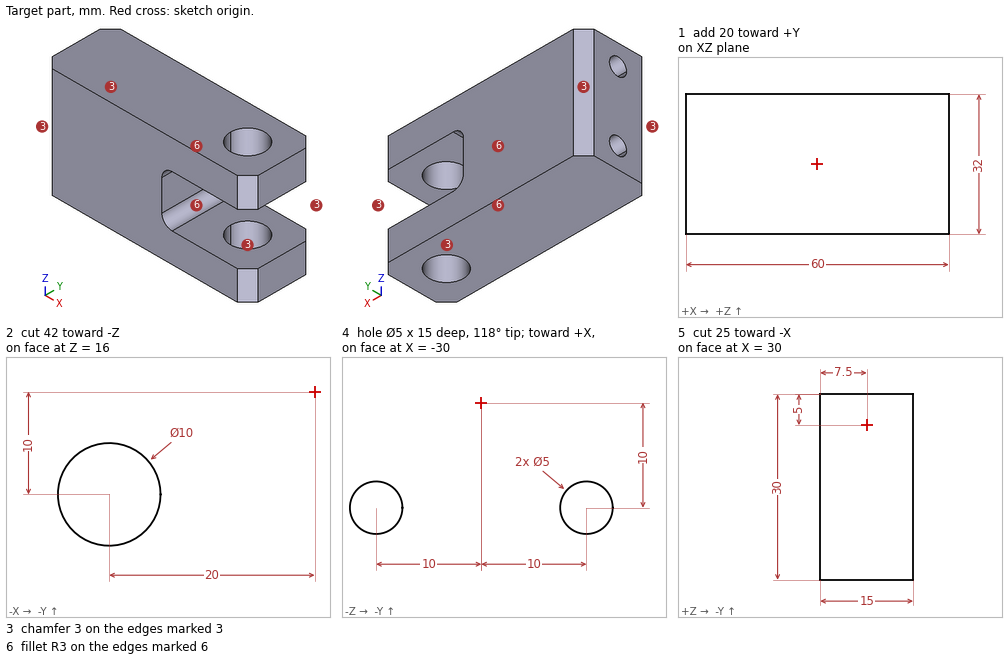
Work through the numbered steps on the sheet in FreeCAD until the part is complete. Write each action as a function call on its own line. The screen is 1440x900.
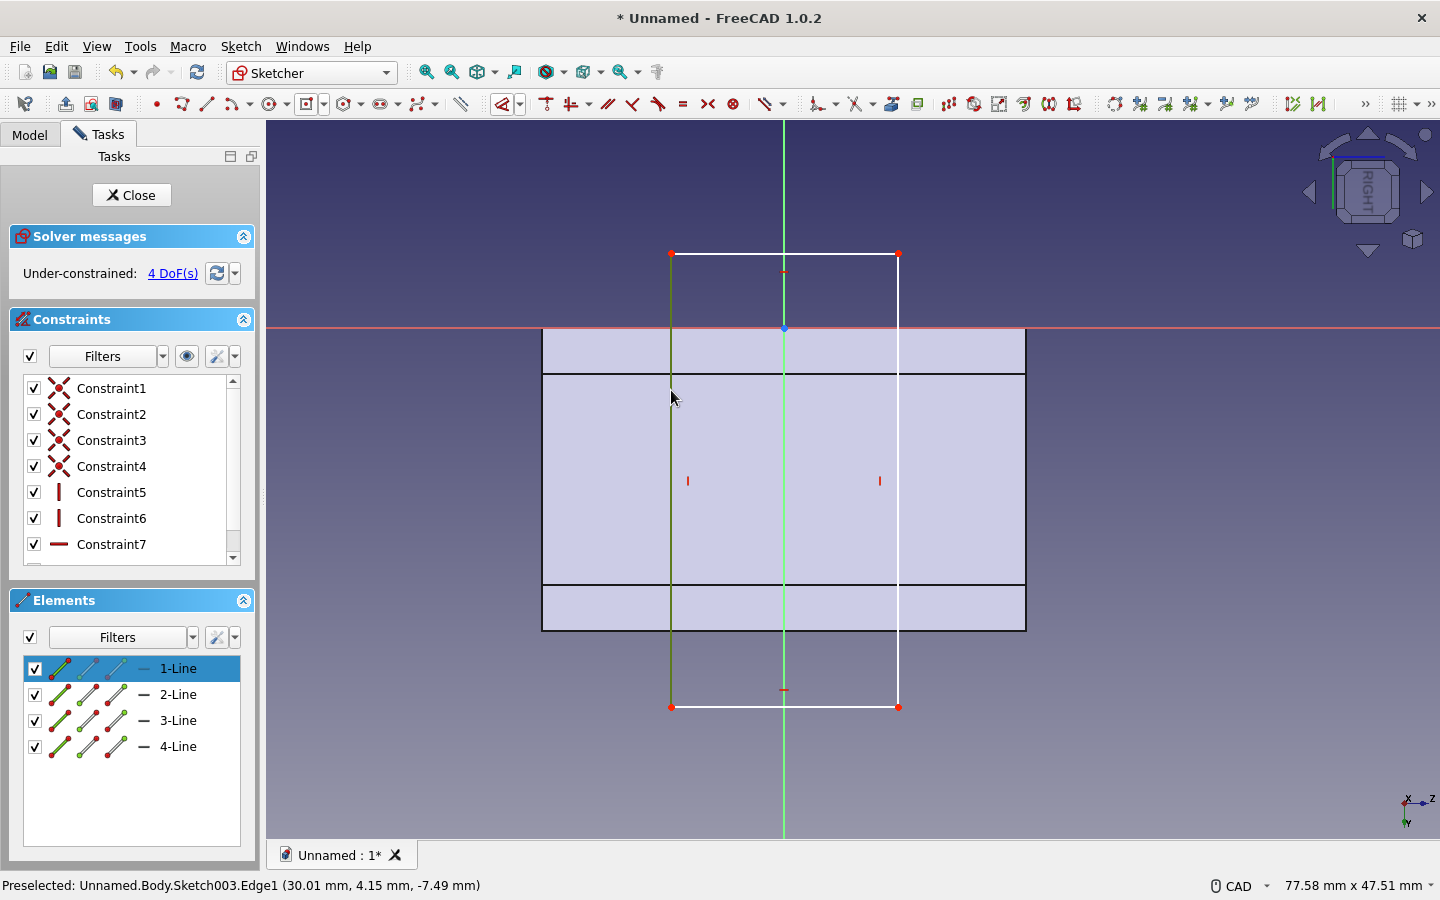
key(i)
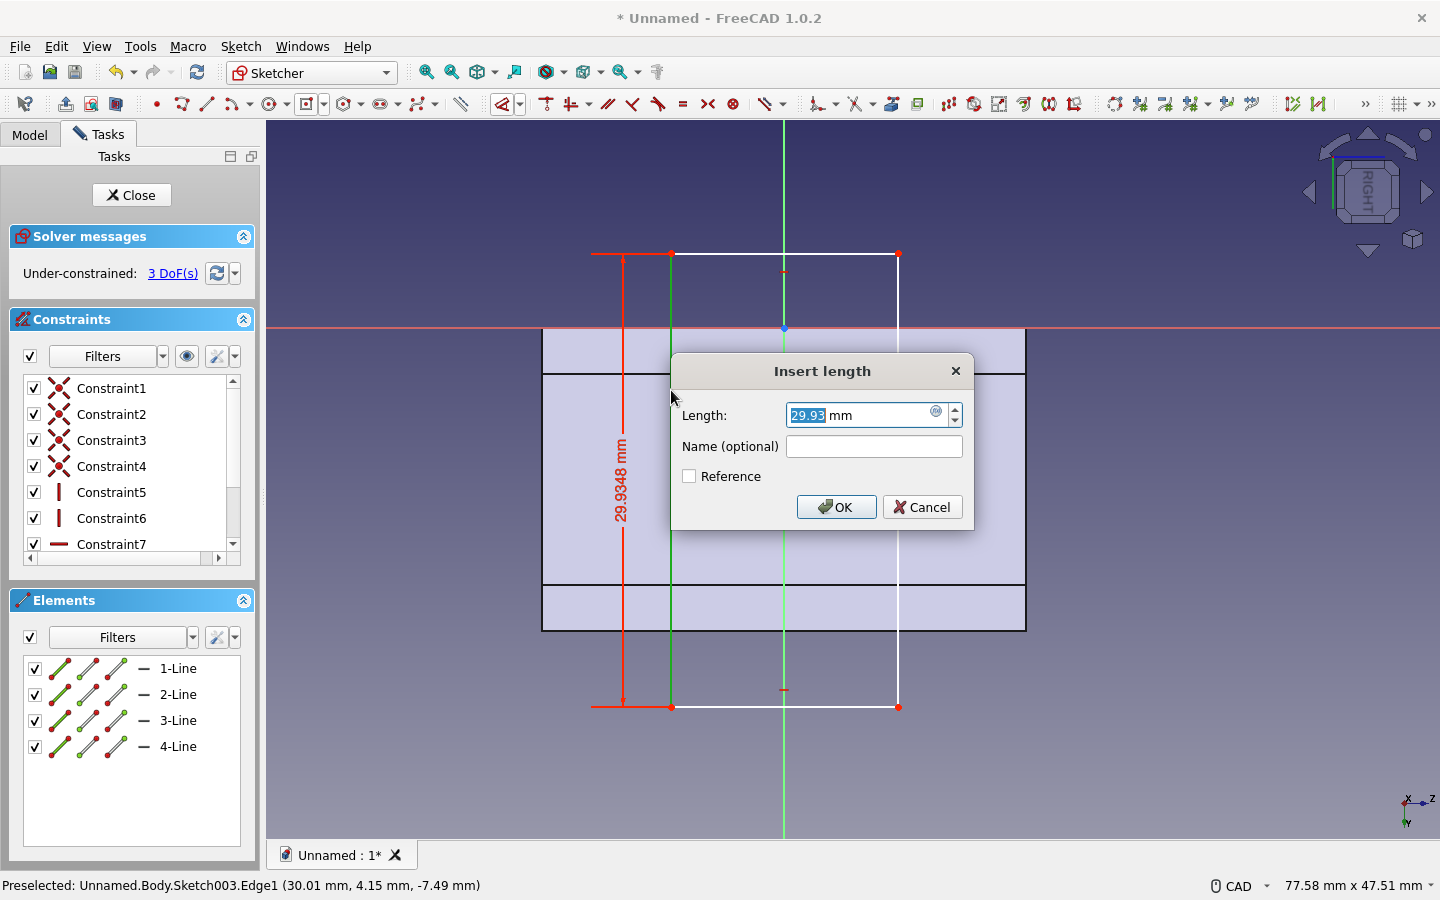
text(30)
key(Return)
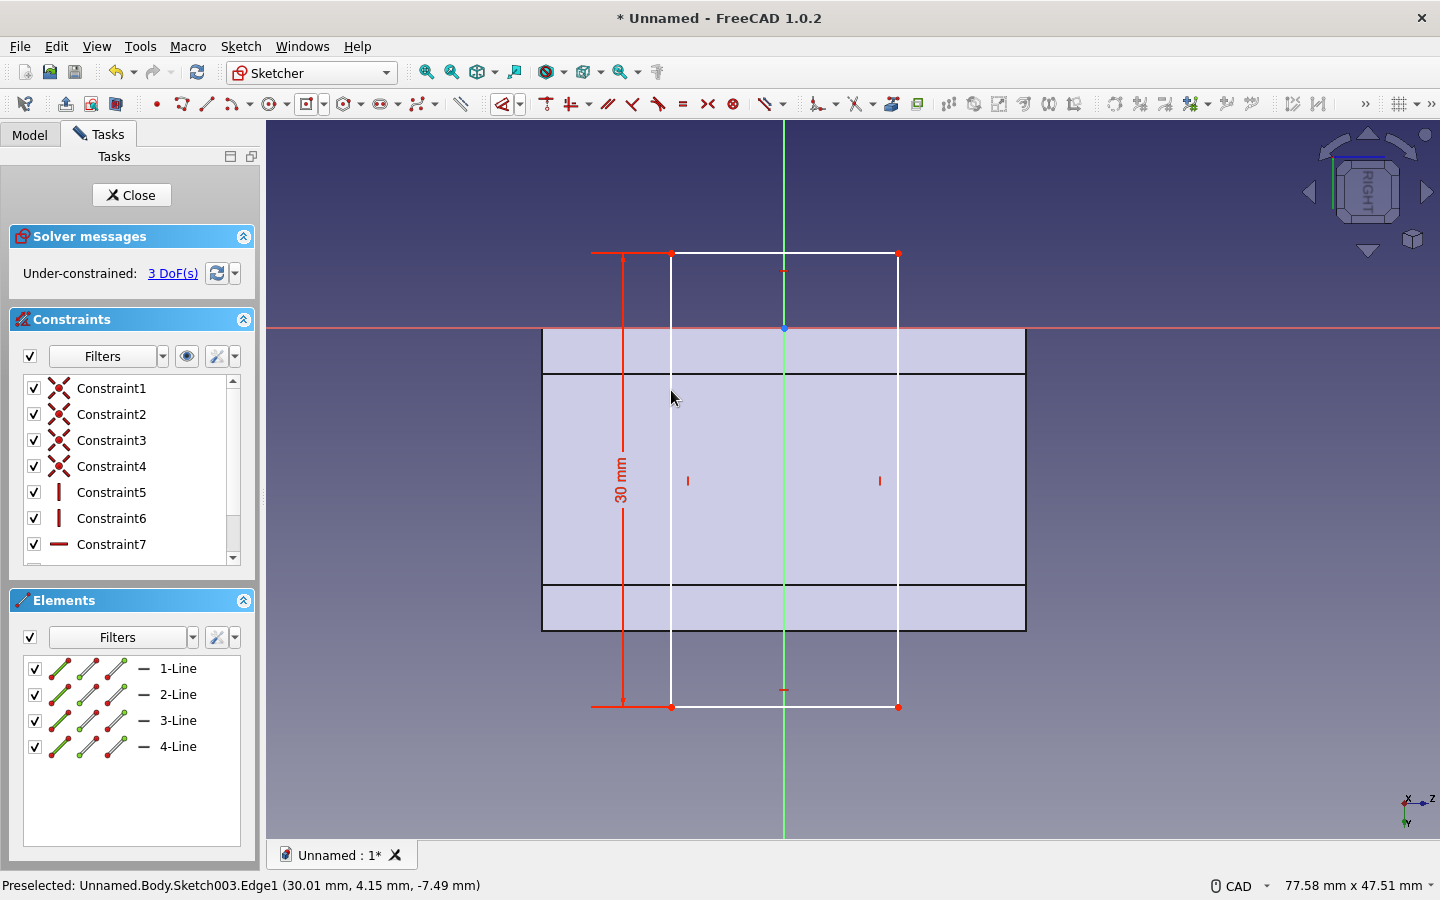
click(739, 707)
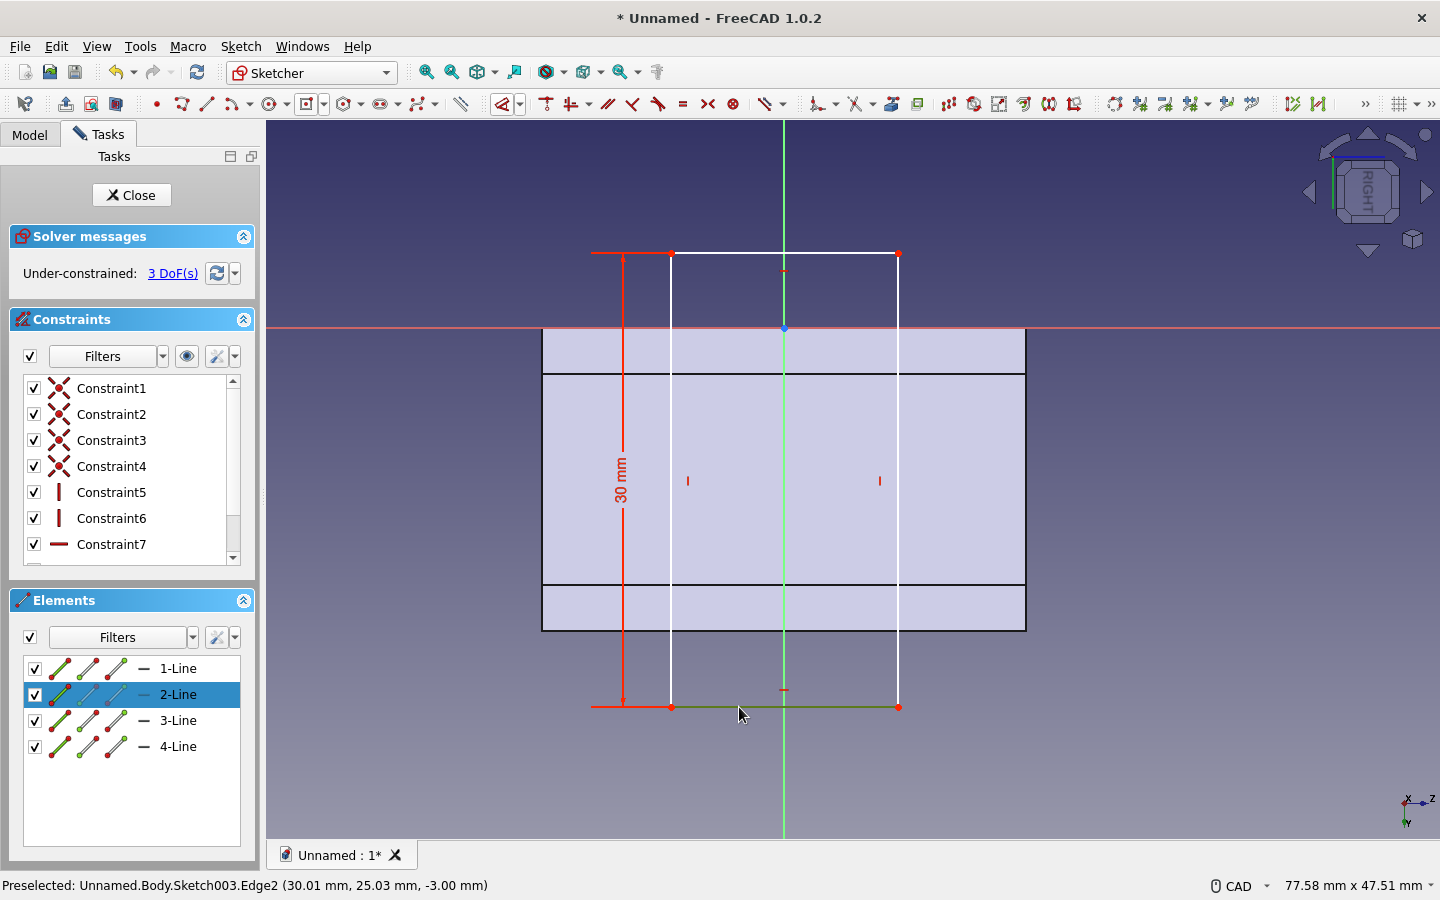
click(520, 104)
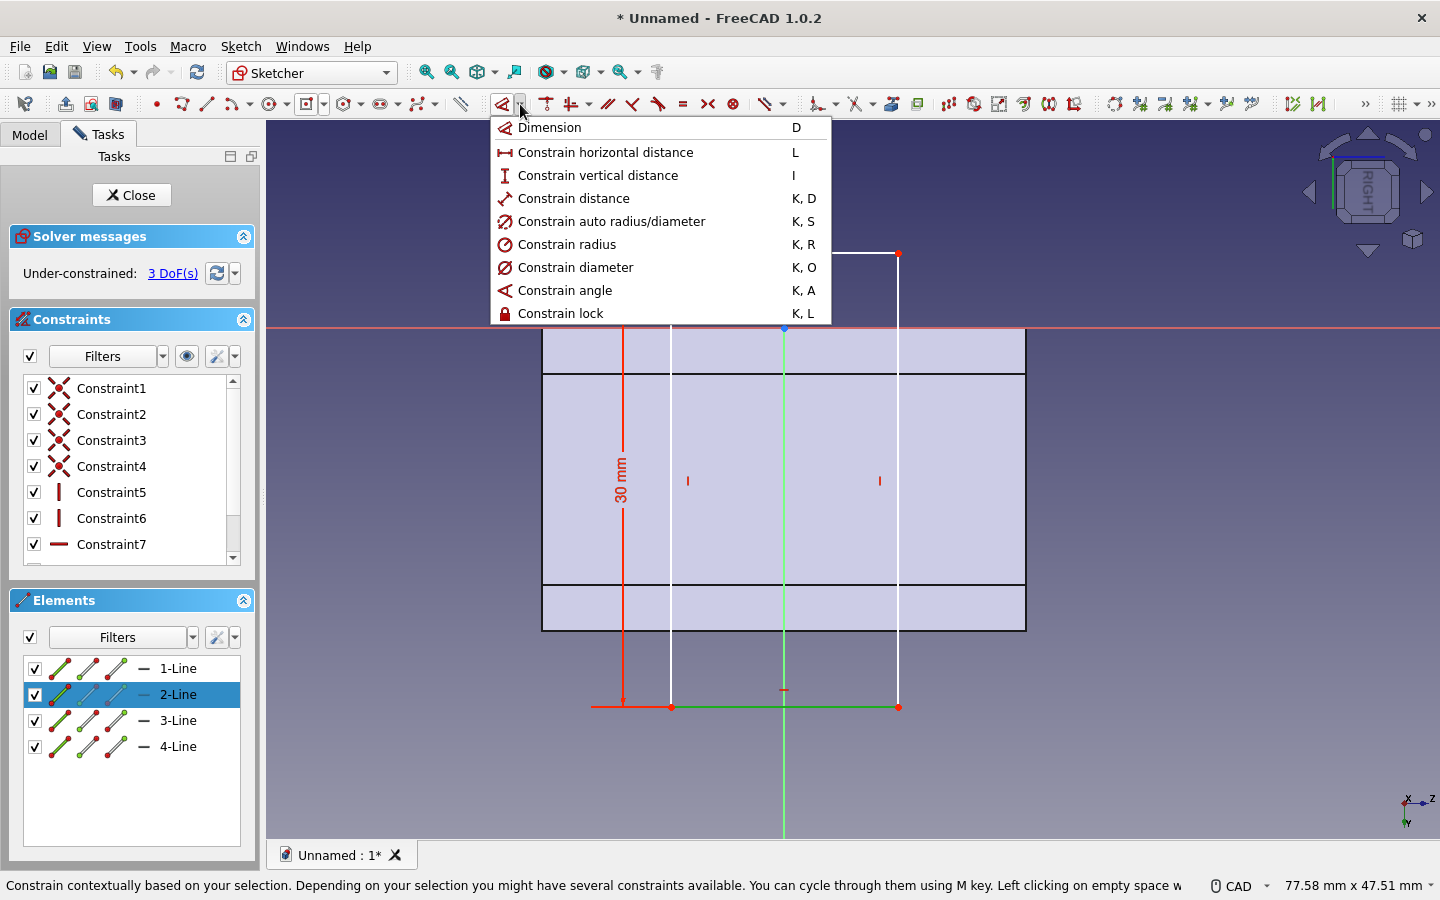
click(661, 152)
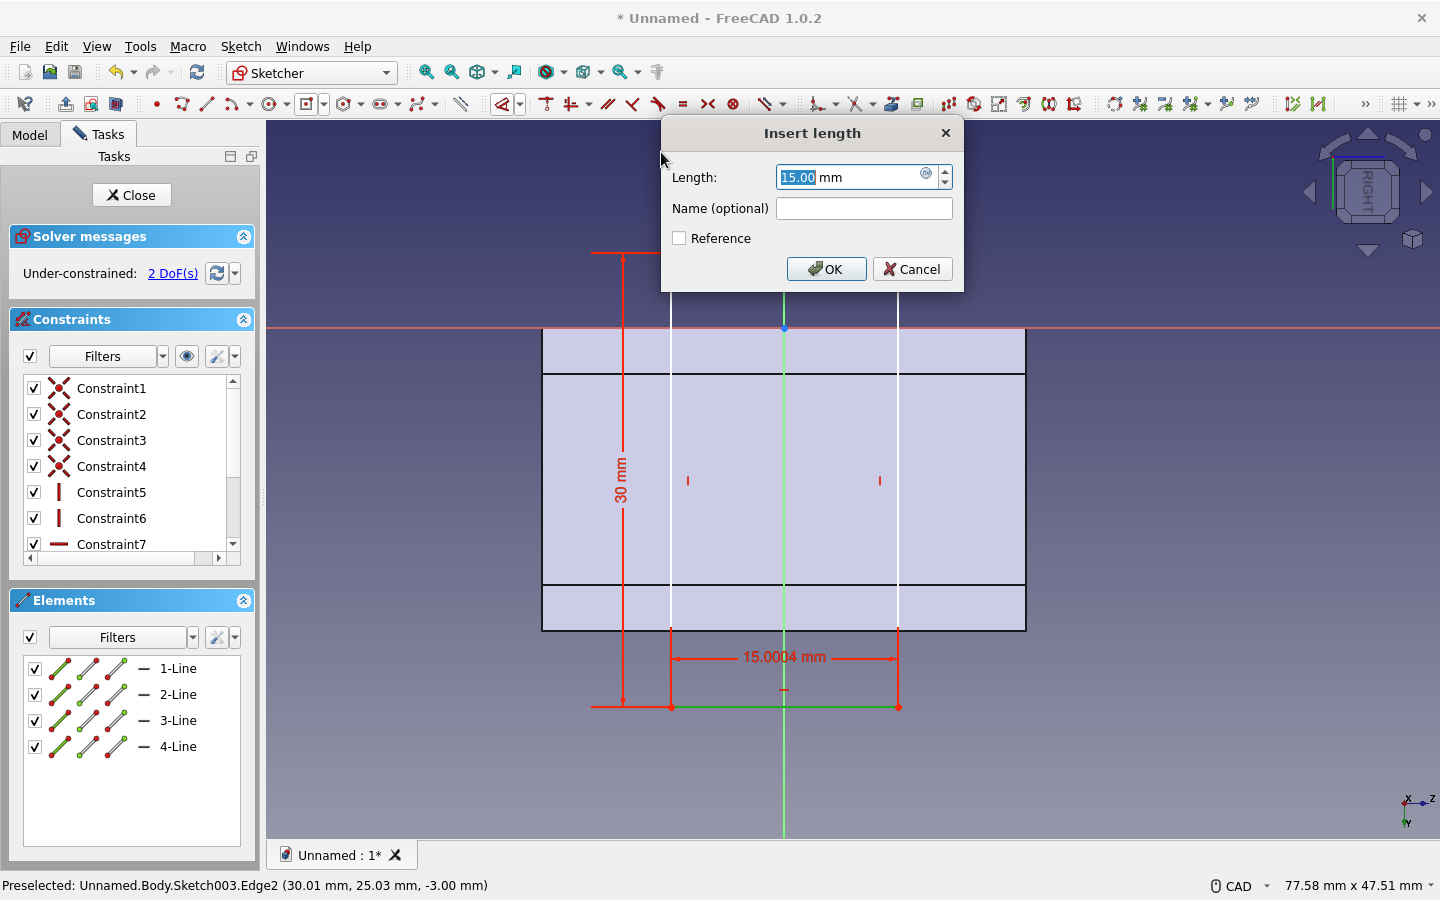
text(15)
key(Return)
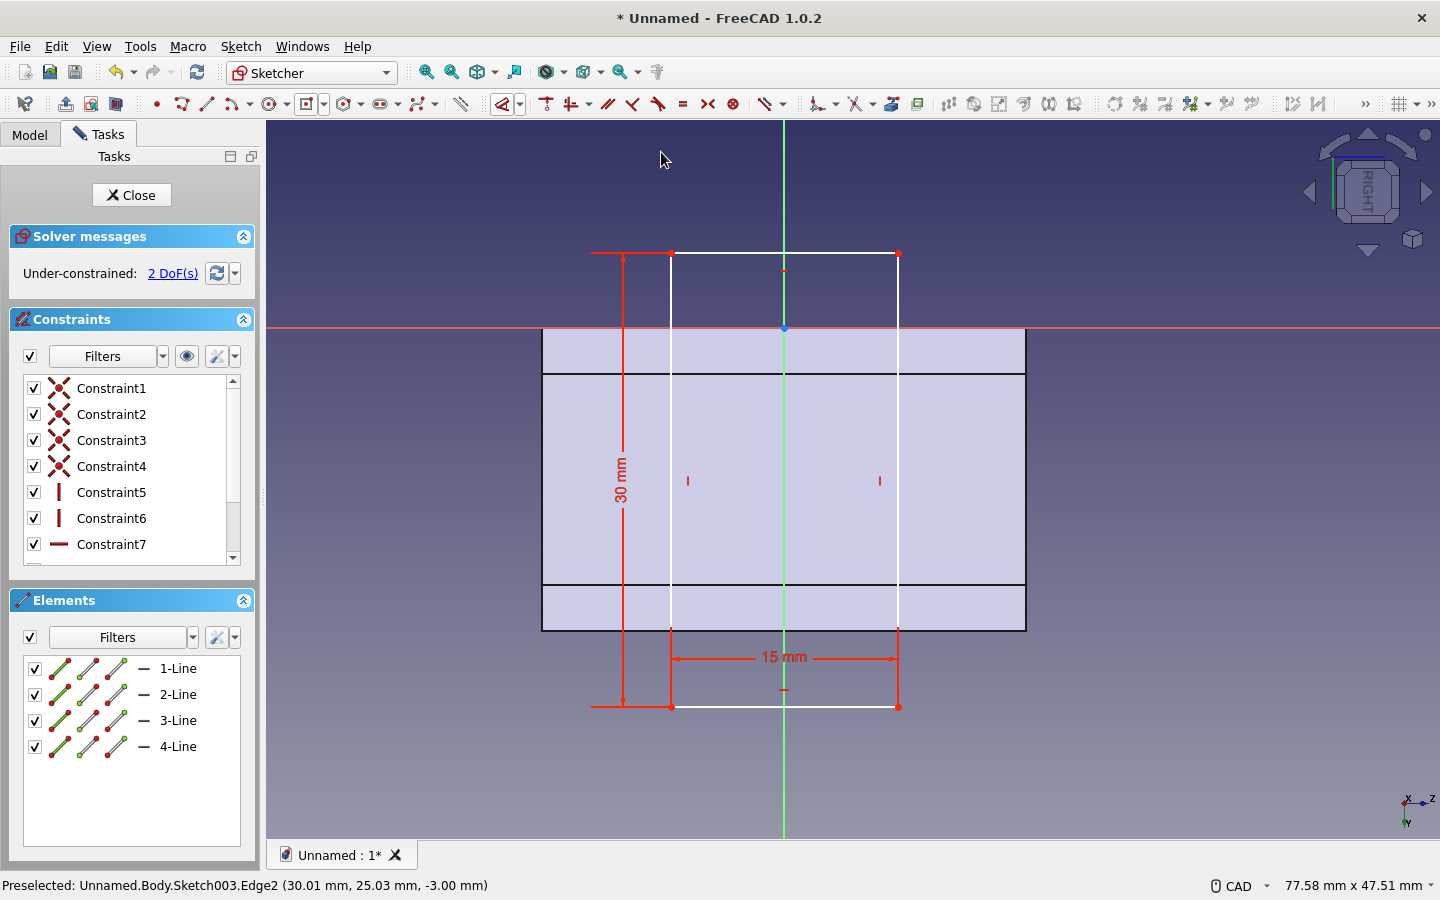
click(671, 253)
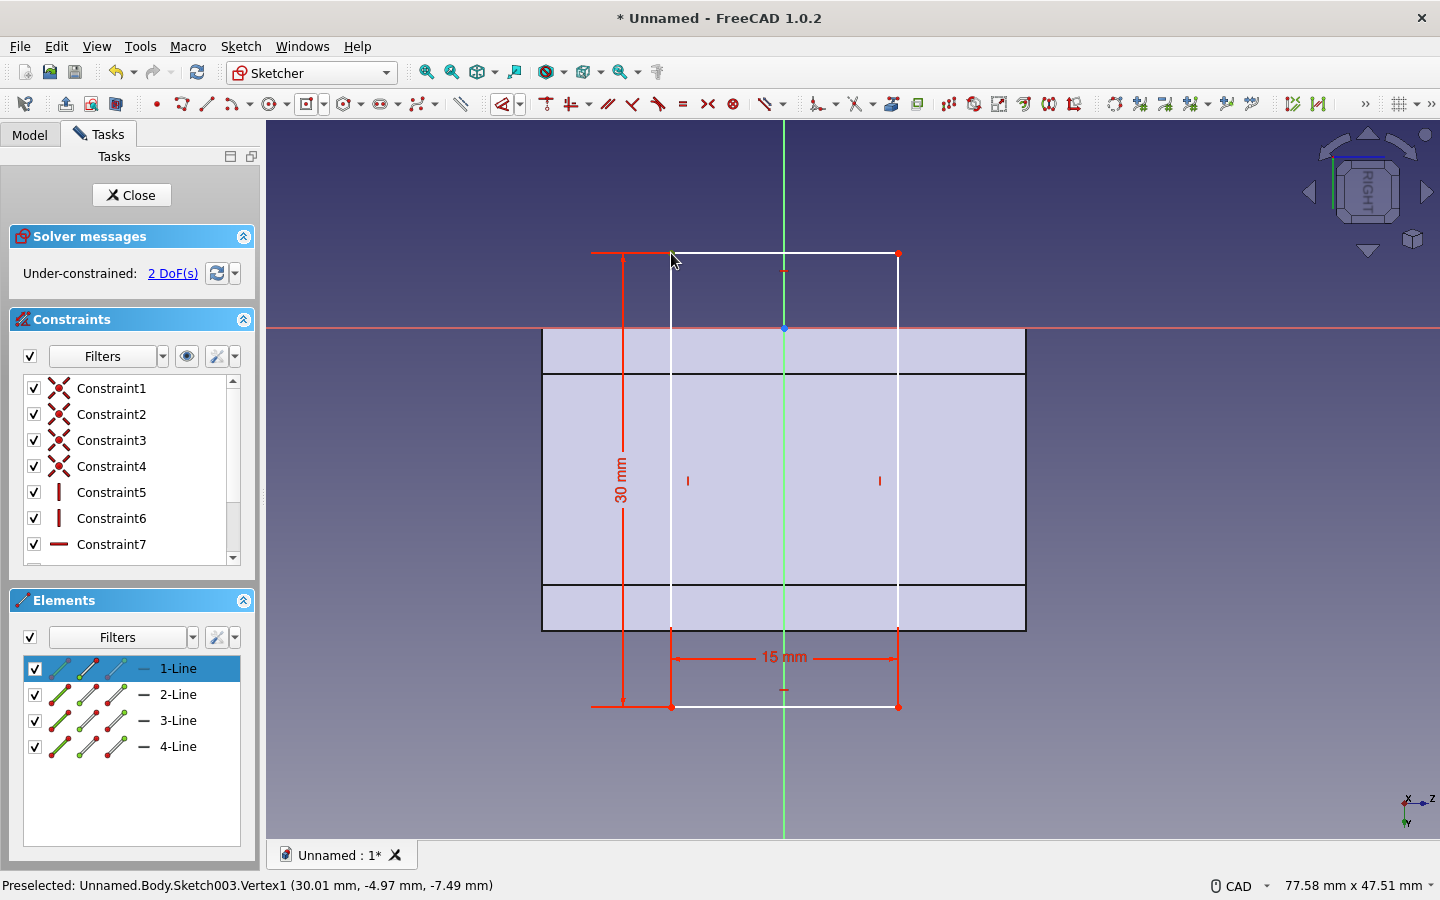
click(520, 104)